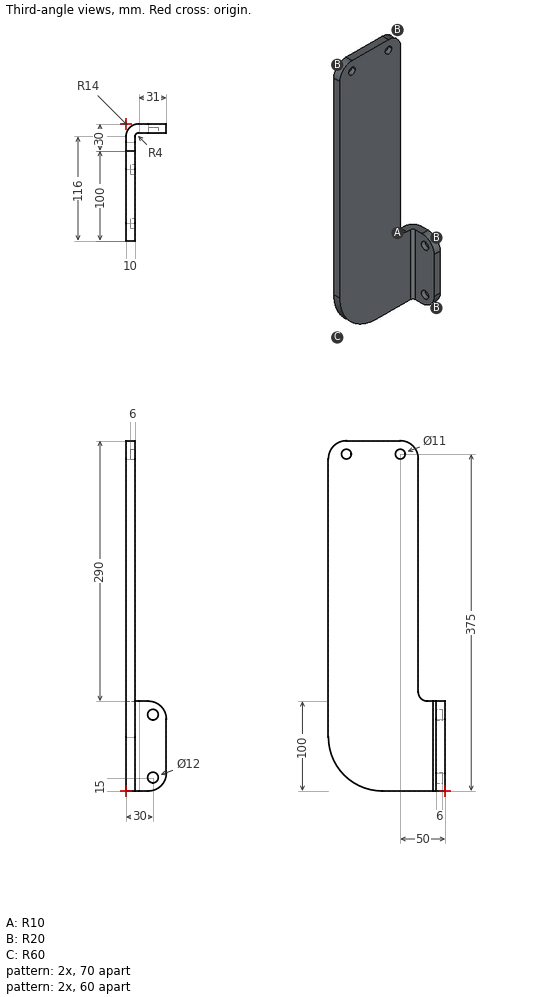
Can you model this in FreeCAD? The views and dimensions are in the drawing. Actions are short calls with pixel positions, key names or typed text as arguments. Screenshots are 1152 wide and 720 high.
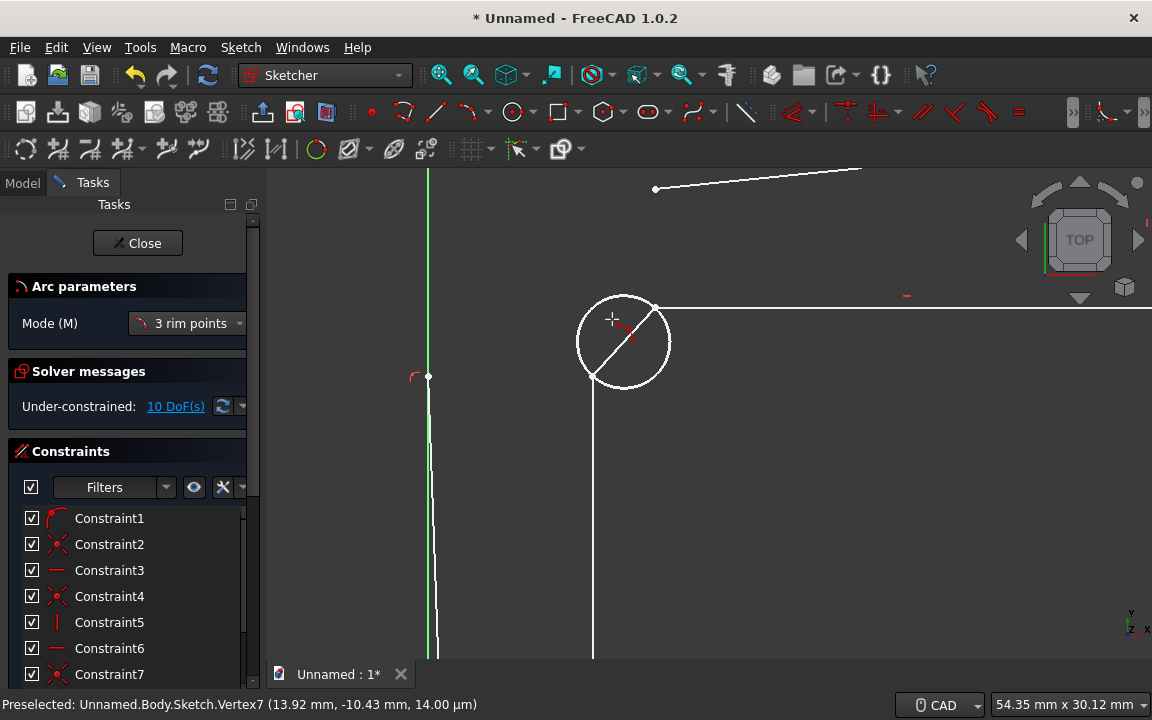
click(610, 320)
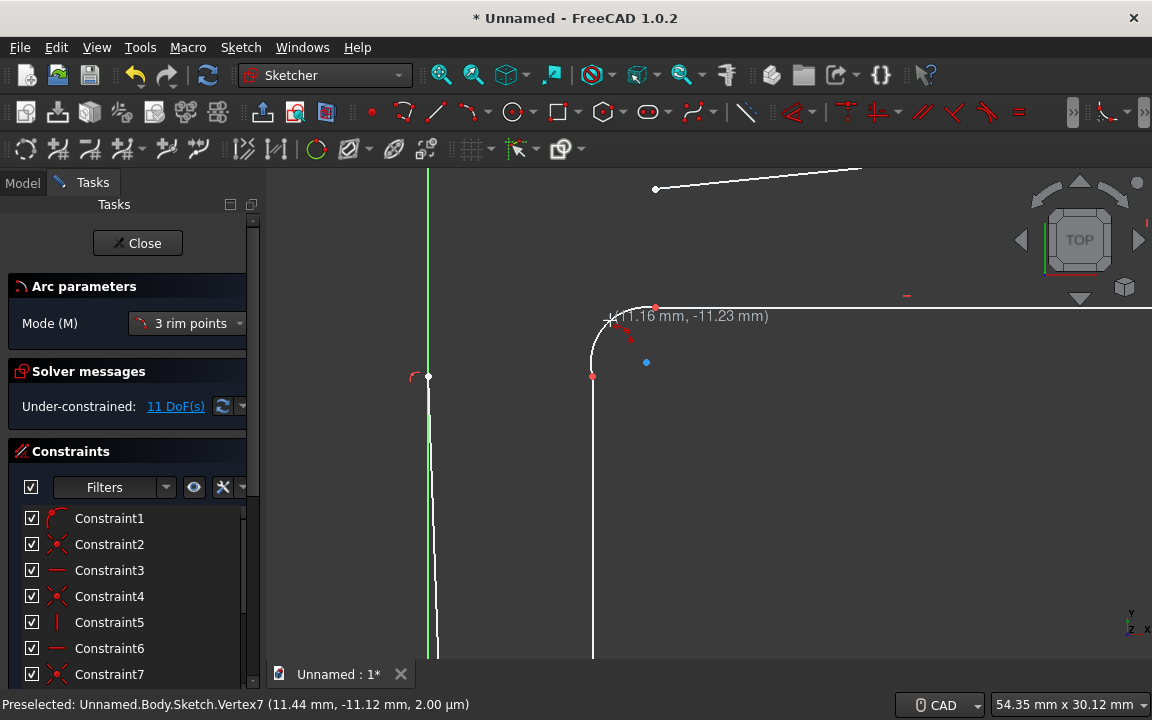
scroll(616, 291, down, 10)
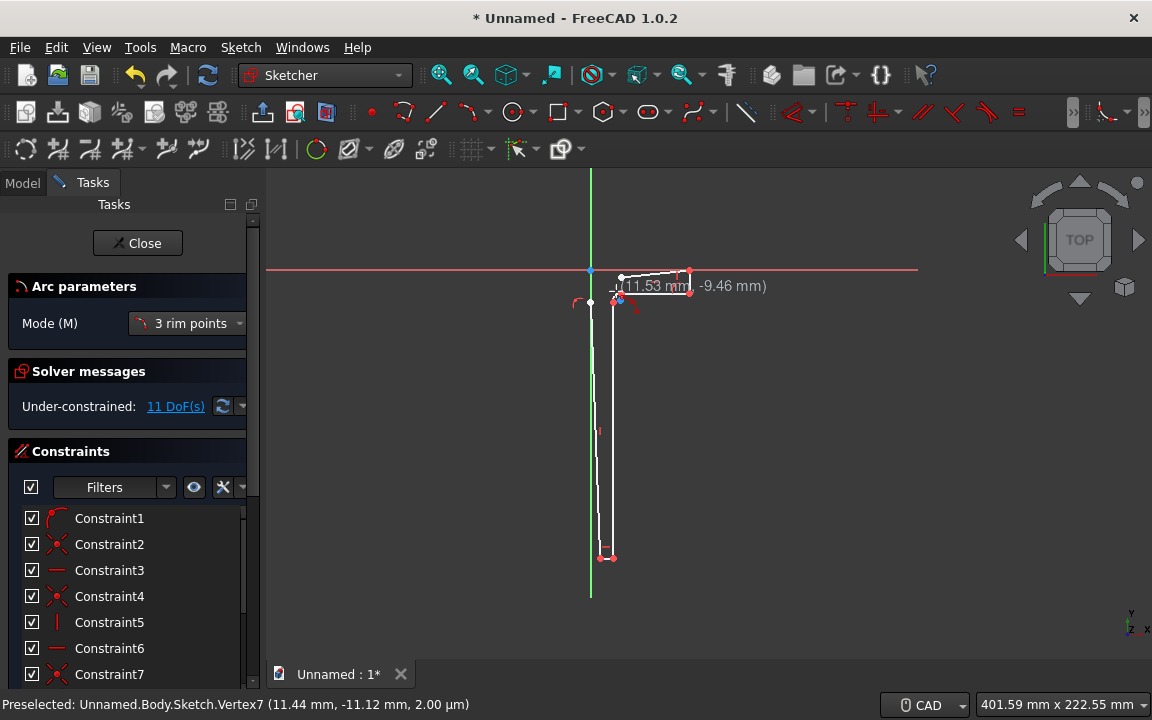
click(622, 277)
click(591, 303)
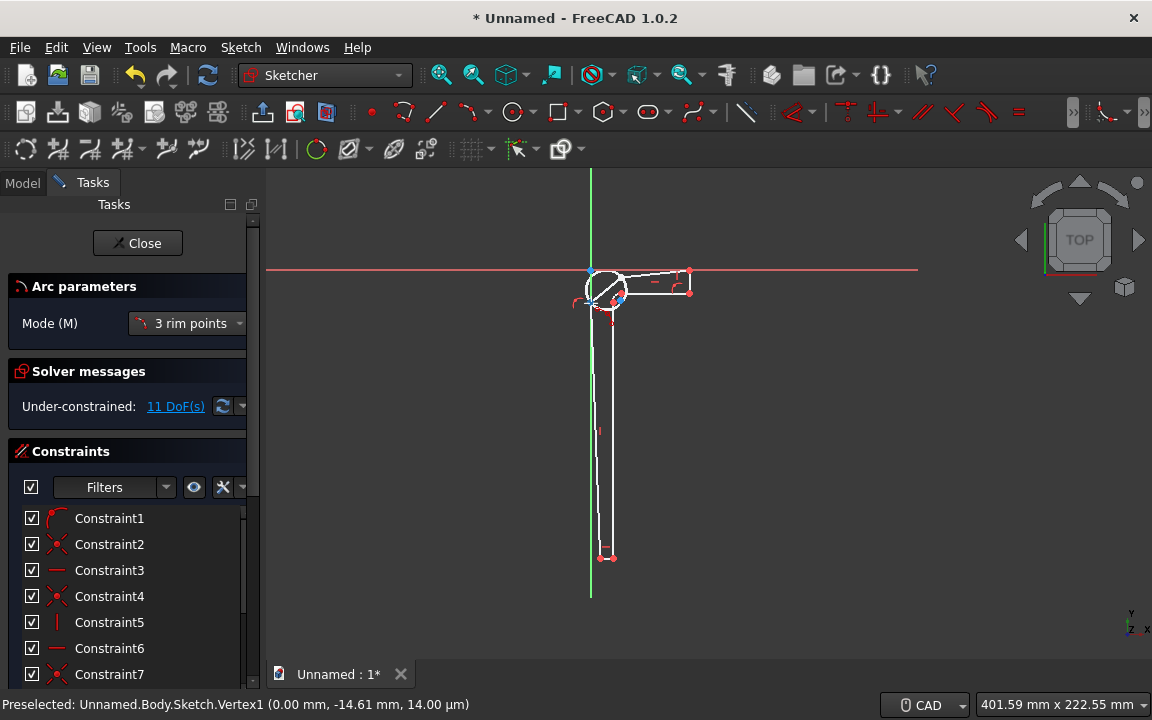
scroll(600, 280, up, 3)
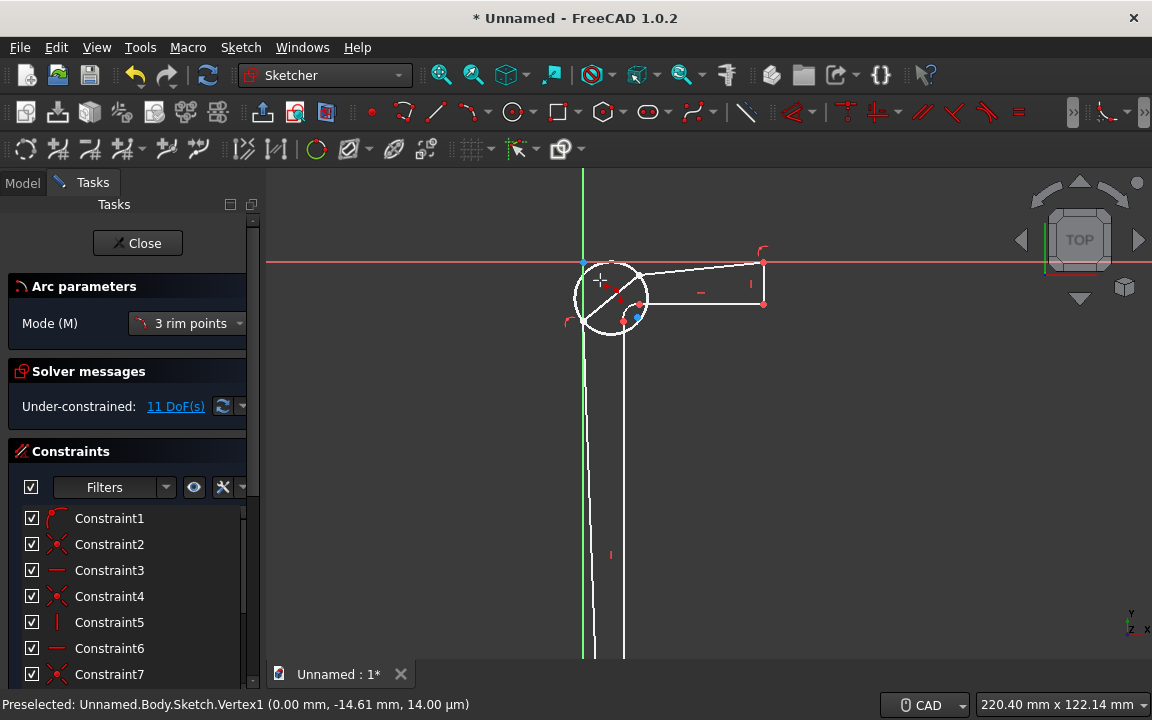
click(600, 279)
key(Escape)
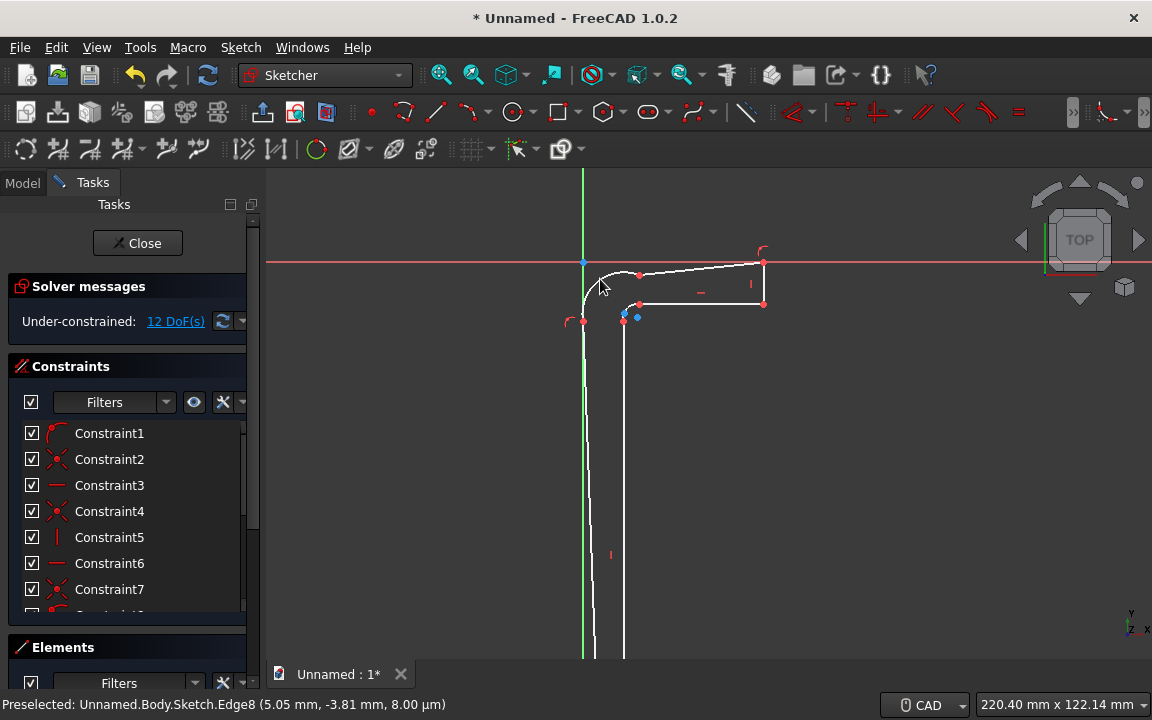
scroll(593, 601, up, 2)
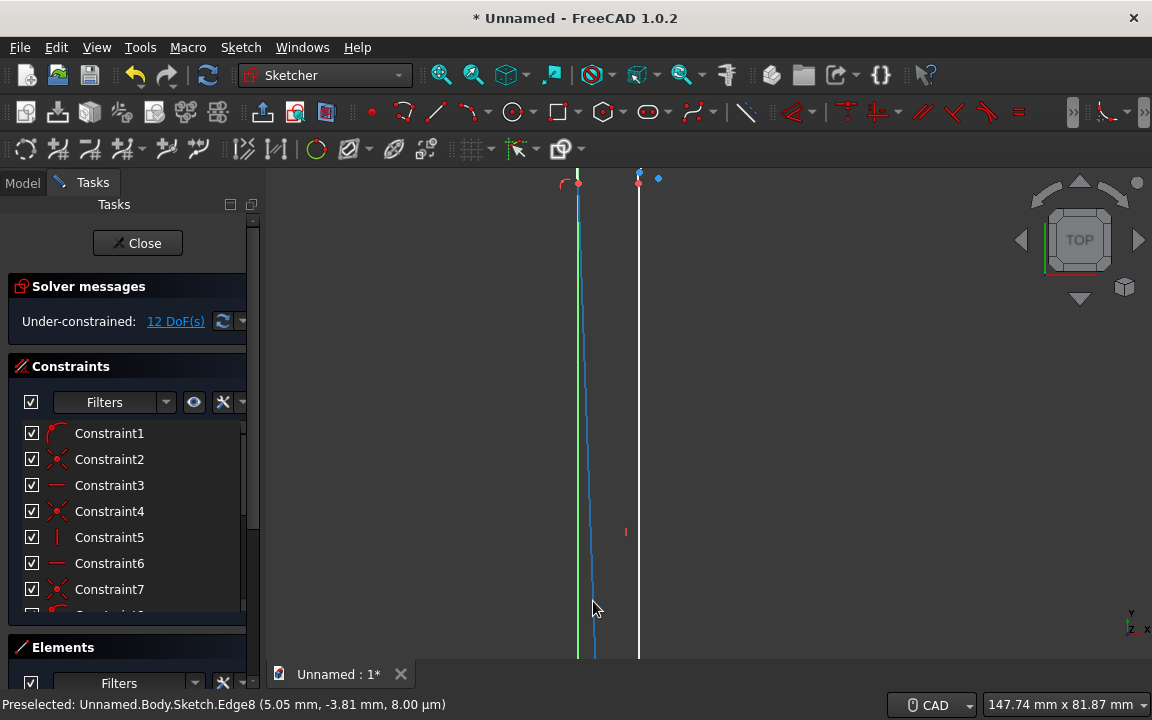
click(593, 601)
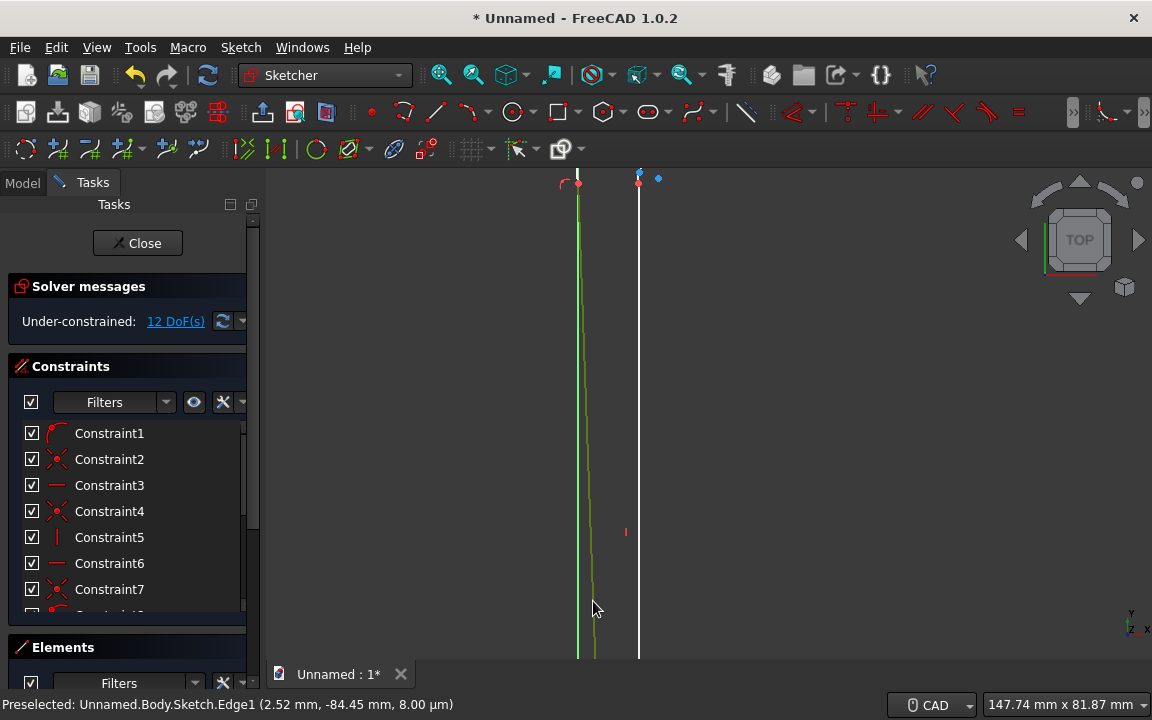
scroll(598, 372, down, 5)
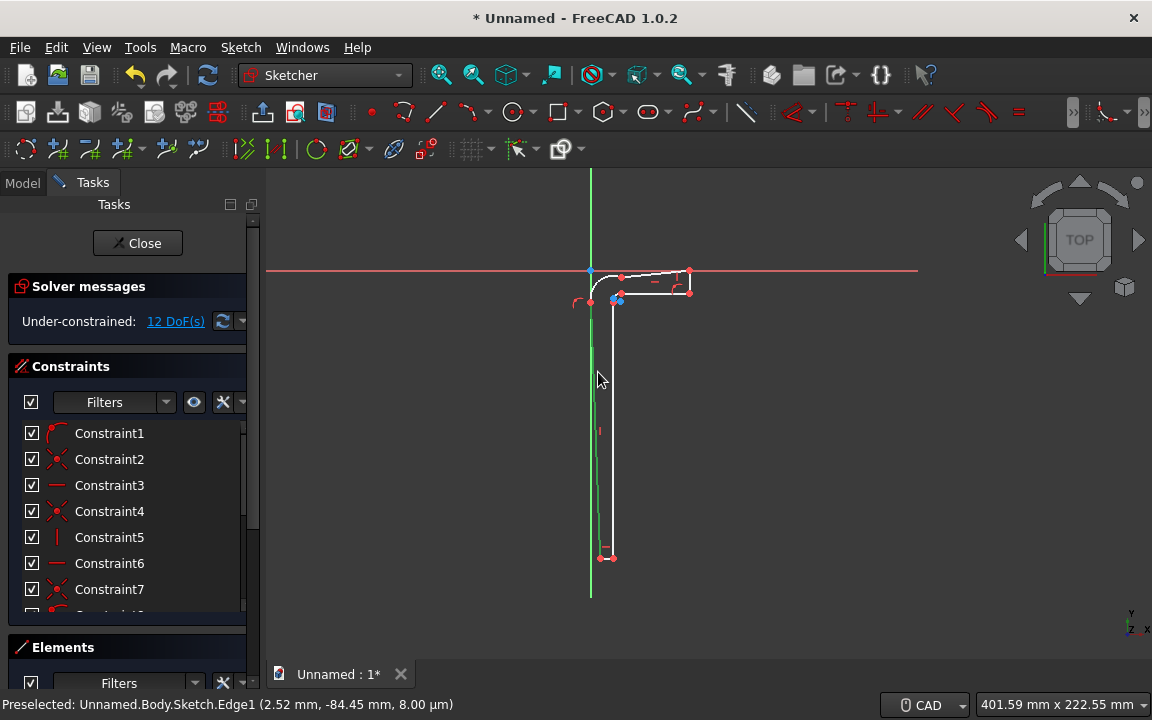
scroll(607, 277, up, 5)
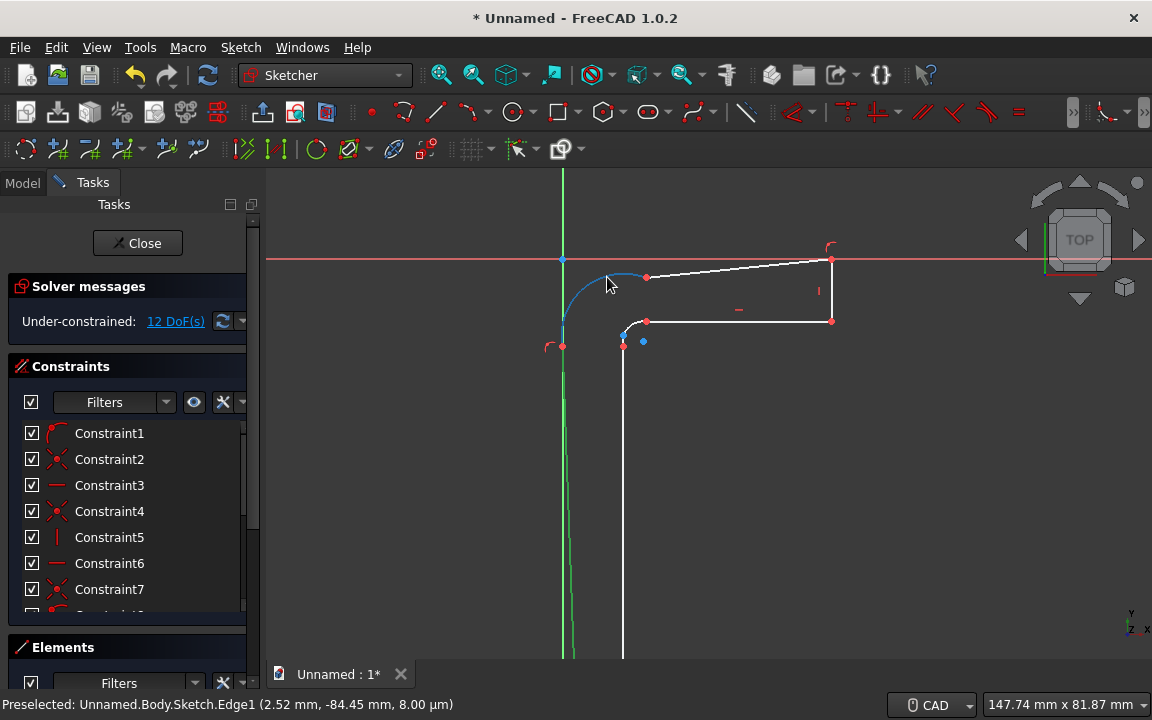
click(607, 276)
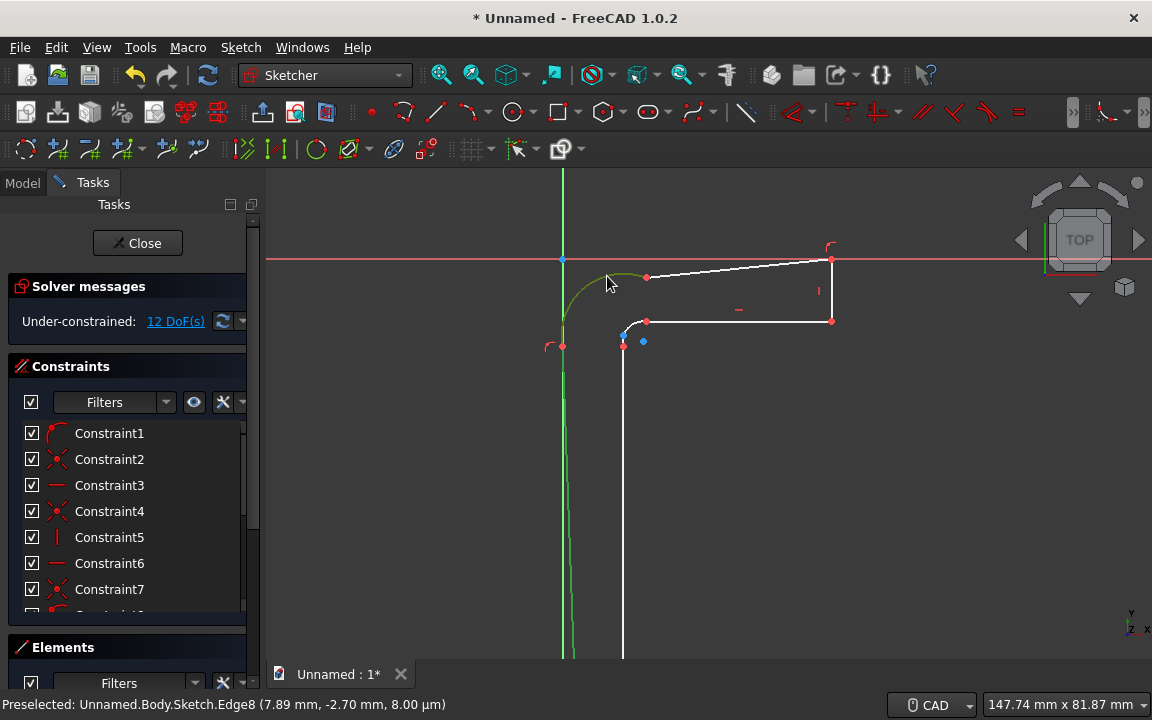
key(t)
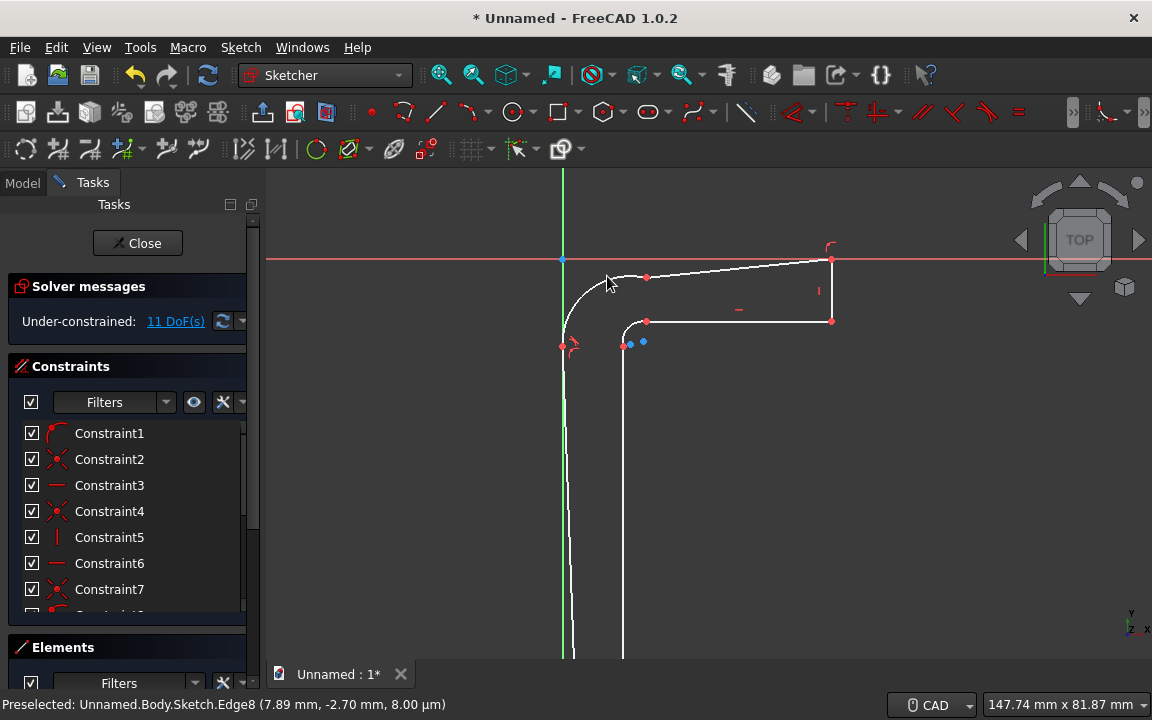
click(623, 556)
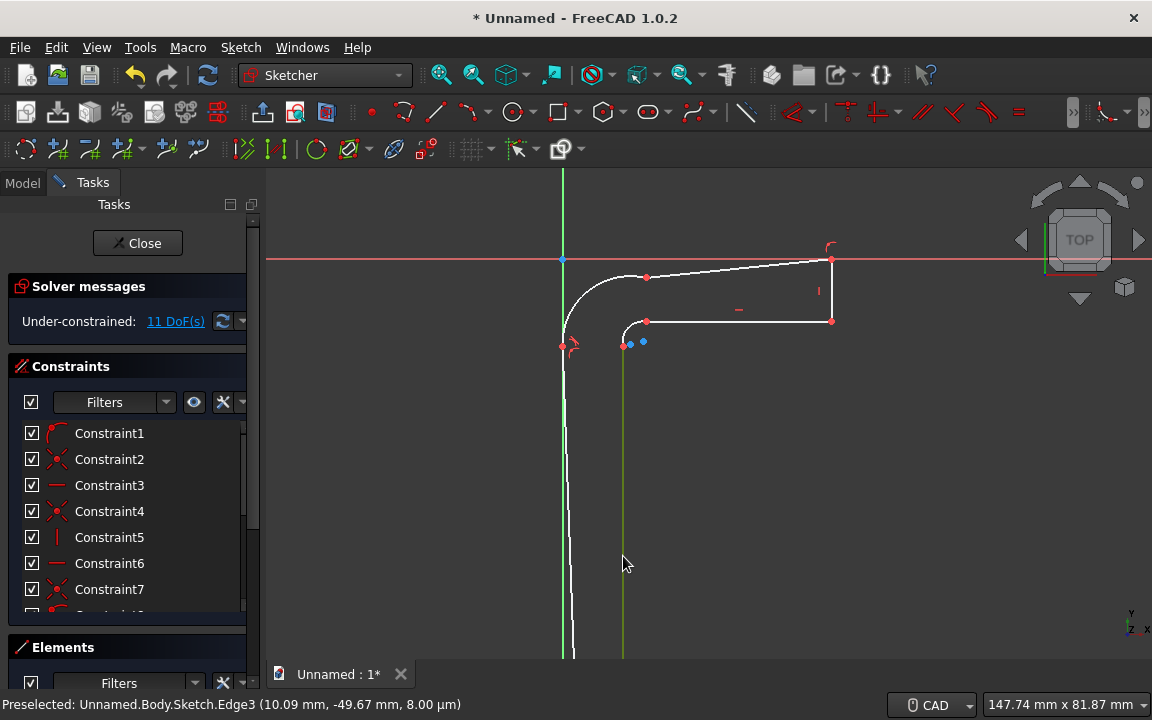
click(634, 323)